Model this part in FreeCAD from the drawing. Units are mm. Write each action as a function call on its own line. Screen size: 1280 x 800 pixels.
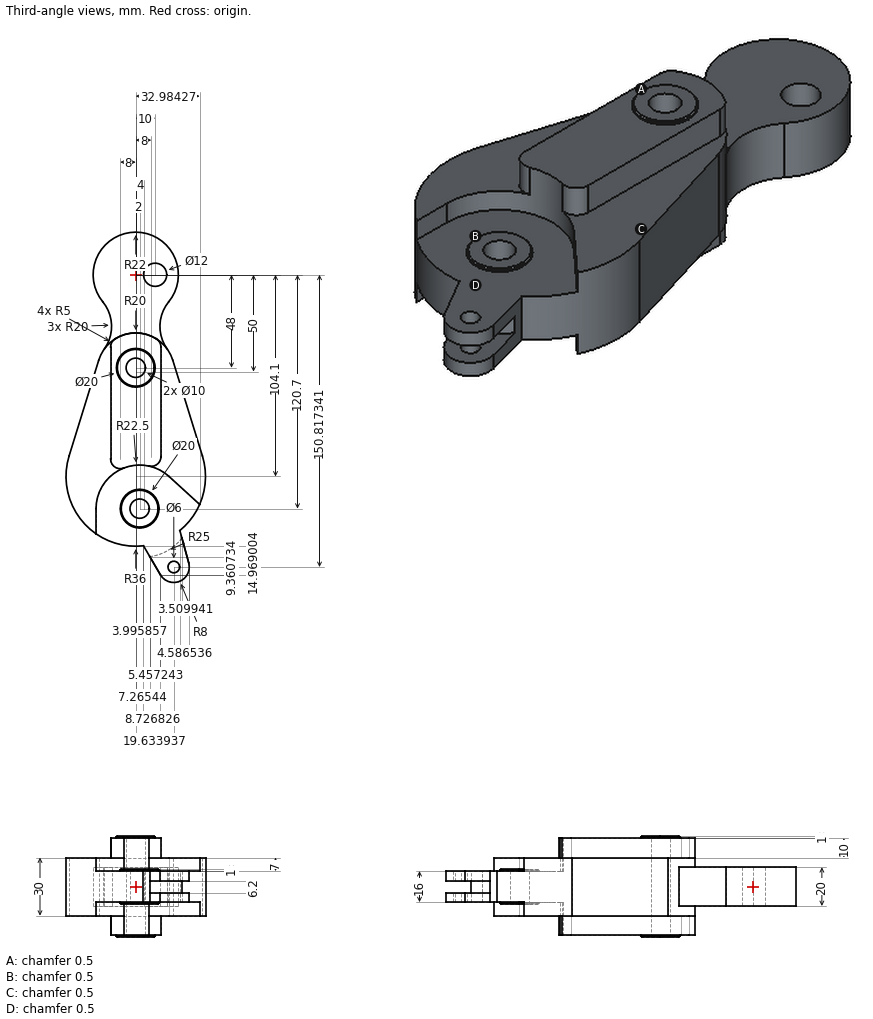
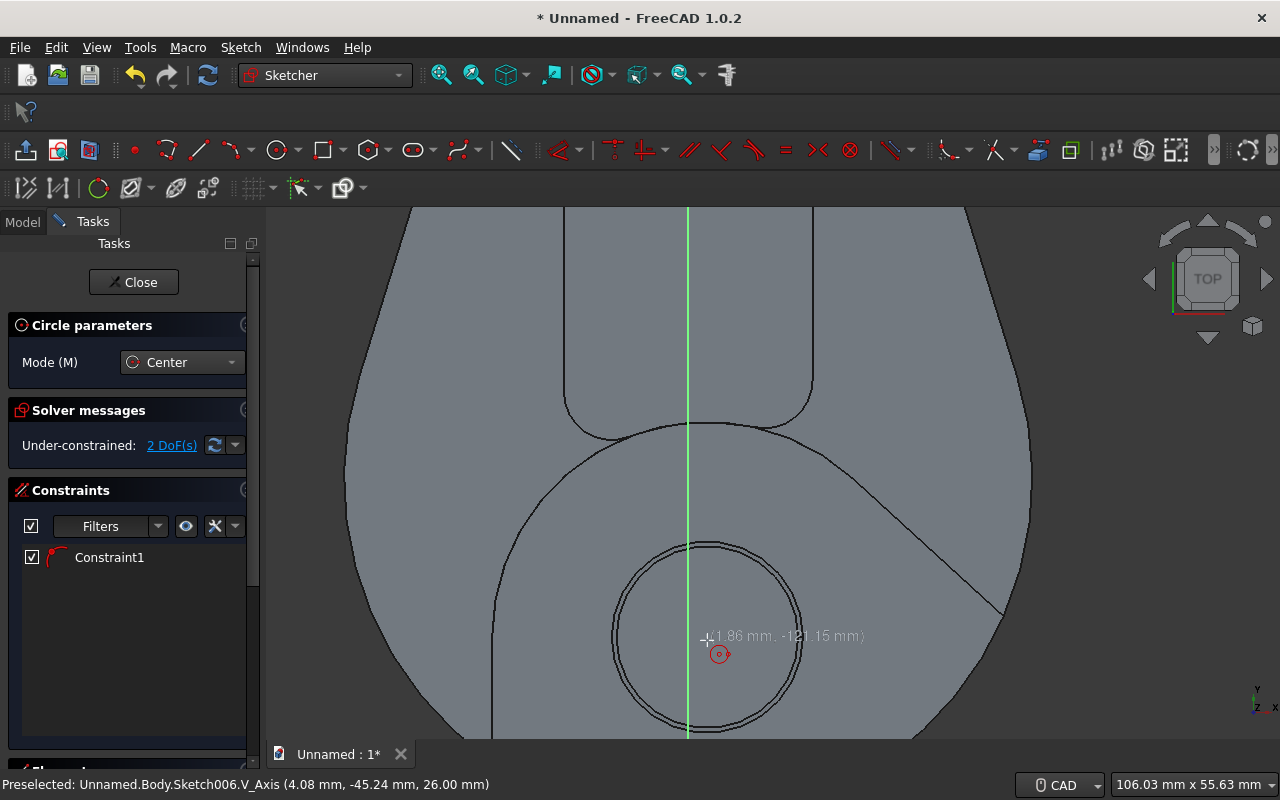
click(707, 637)
click(741, 603)
key(Escape)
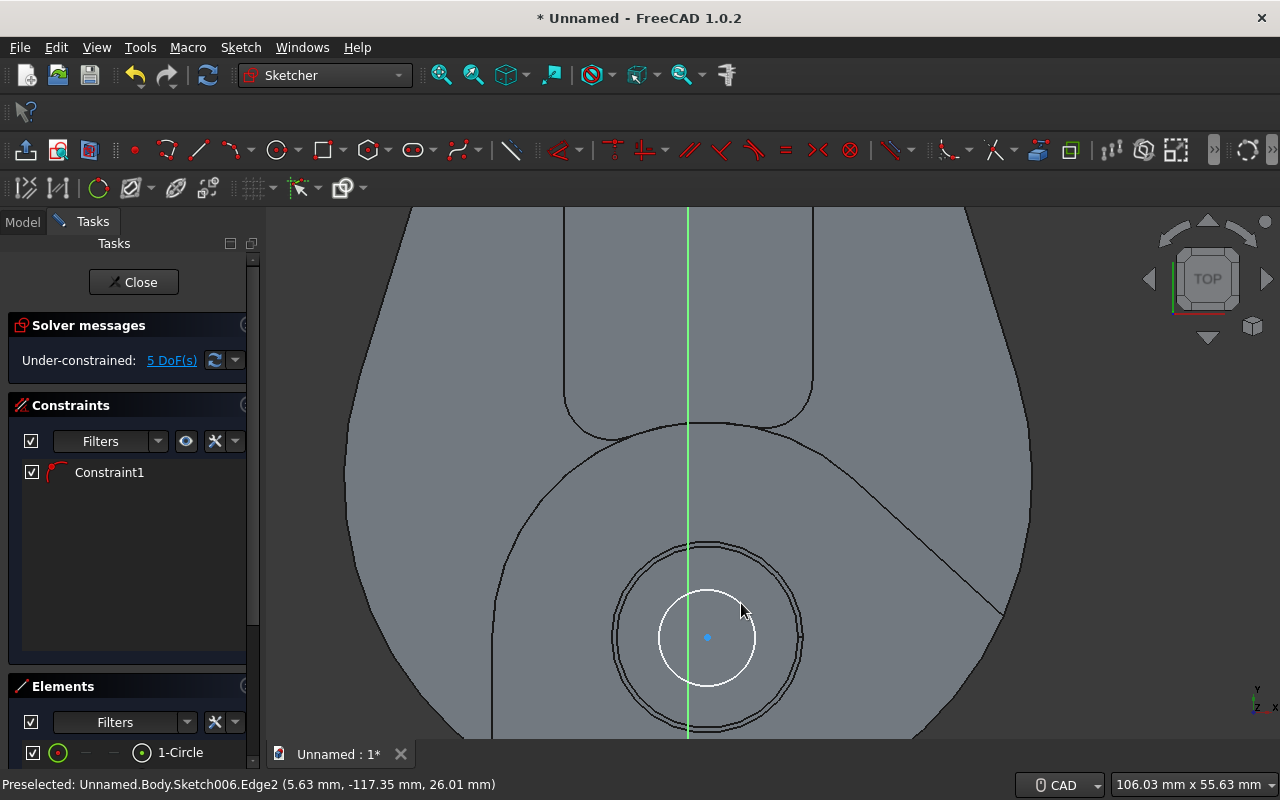
scroll(707, 641, down, 6)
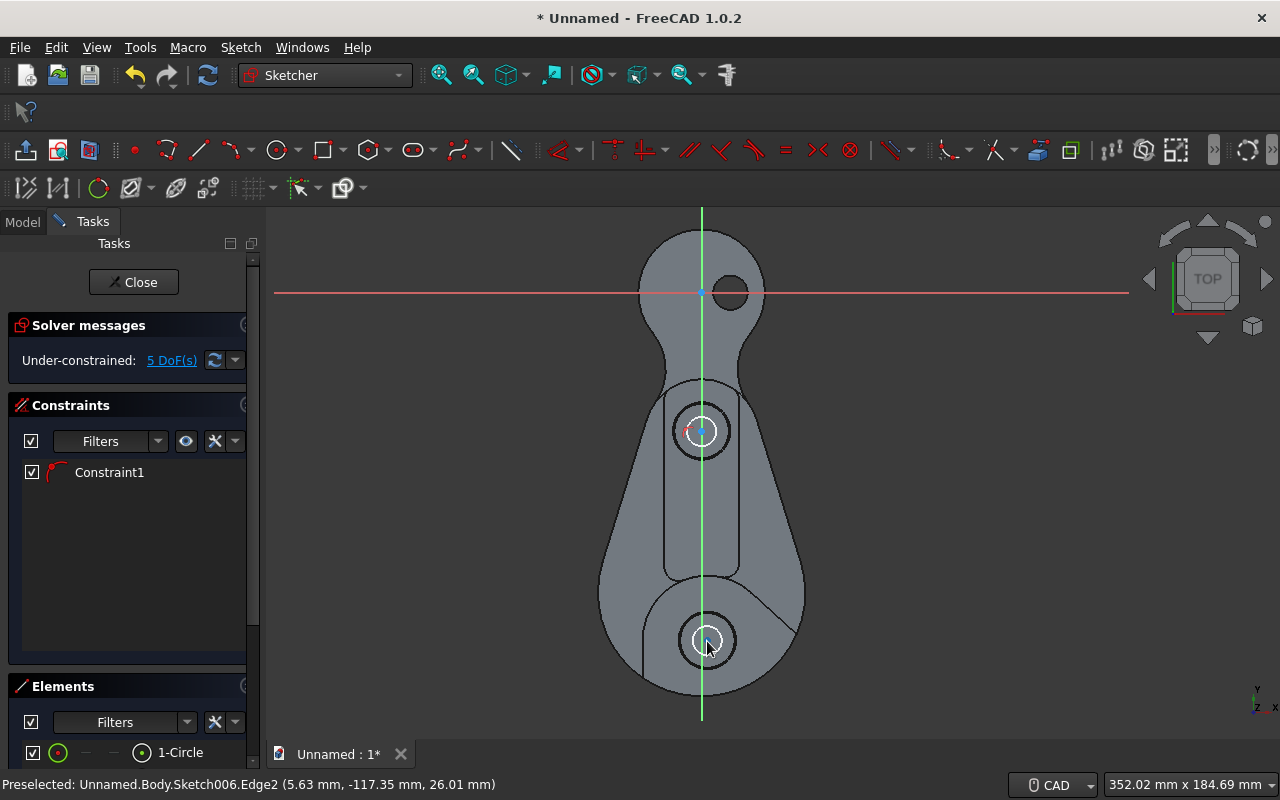
scroll(712, 421, up, 2)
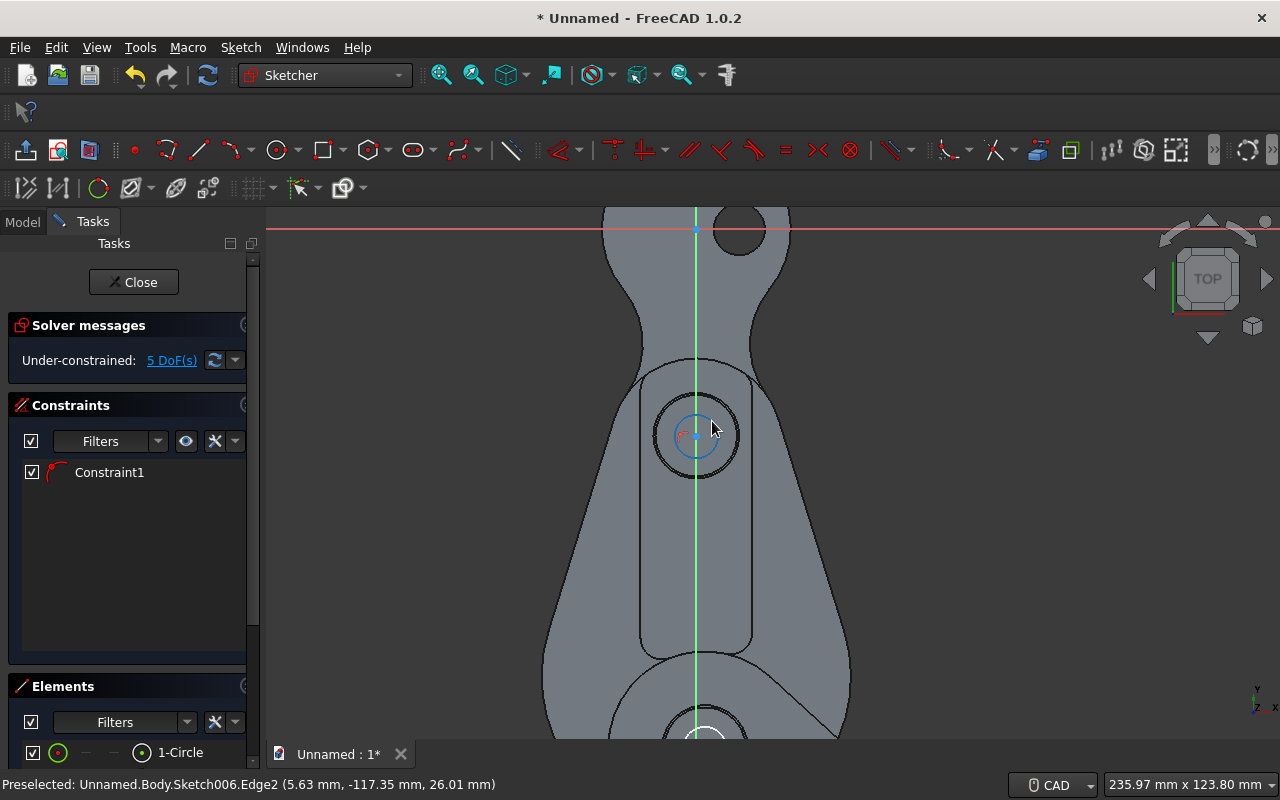
click(712, 421)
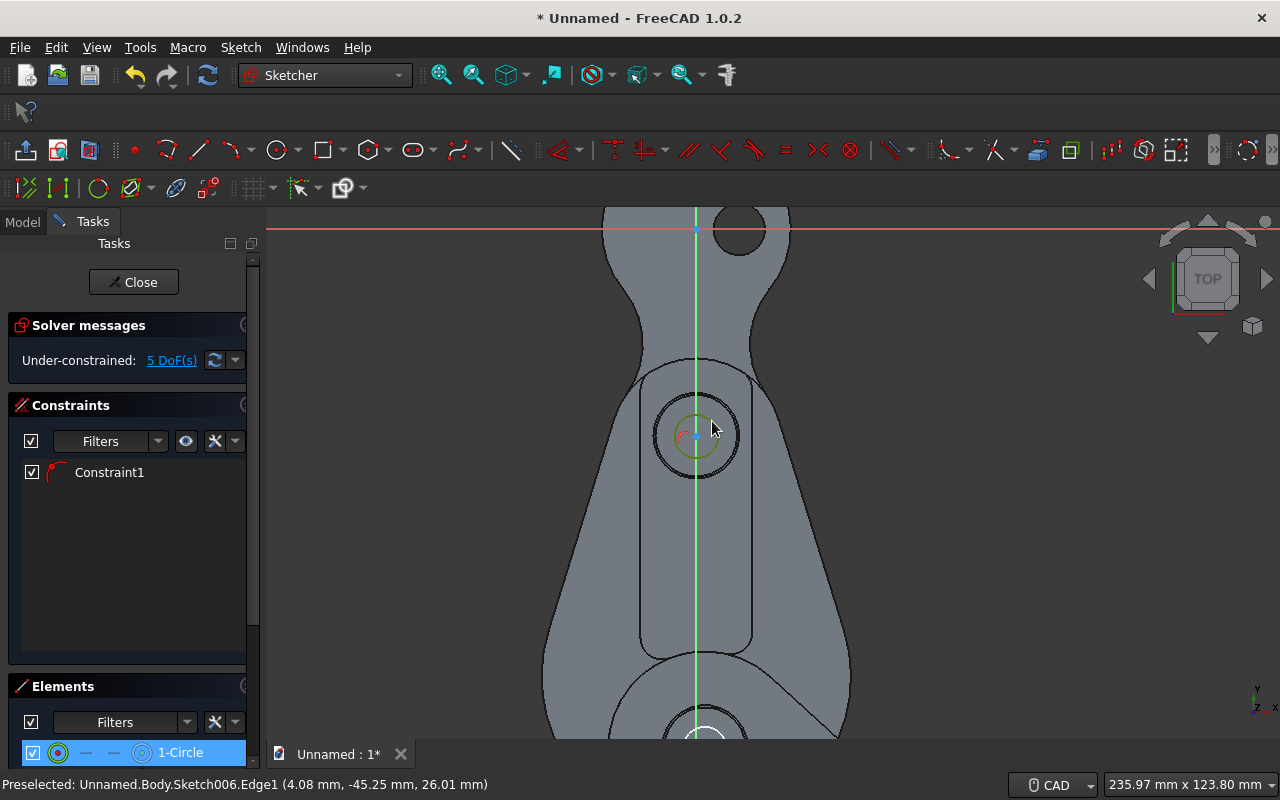
scroll(712, 419, down, 2)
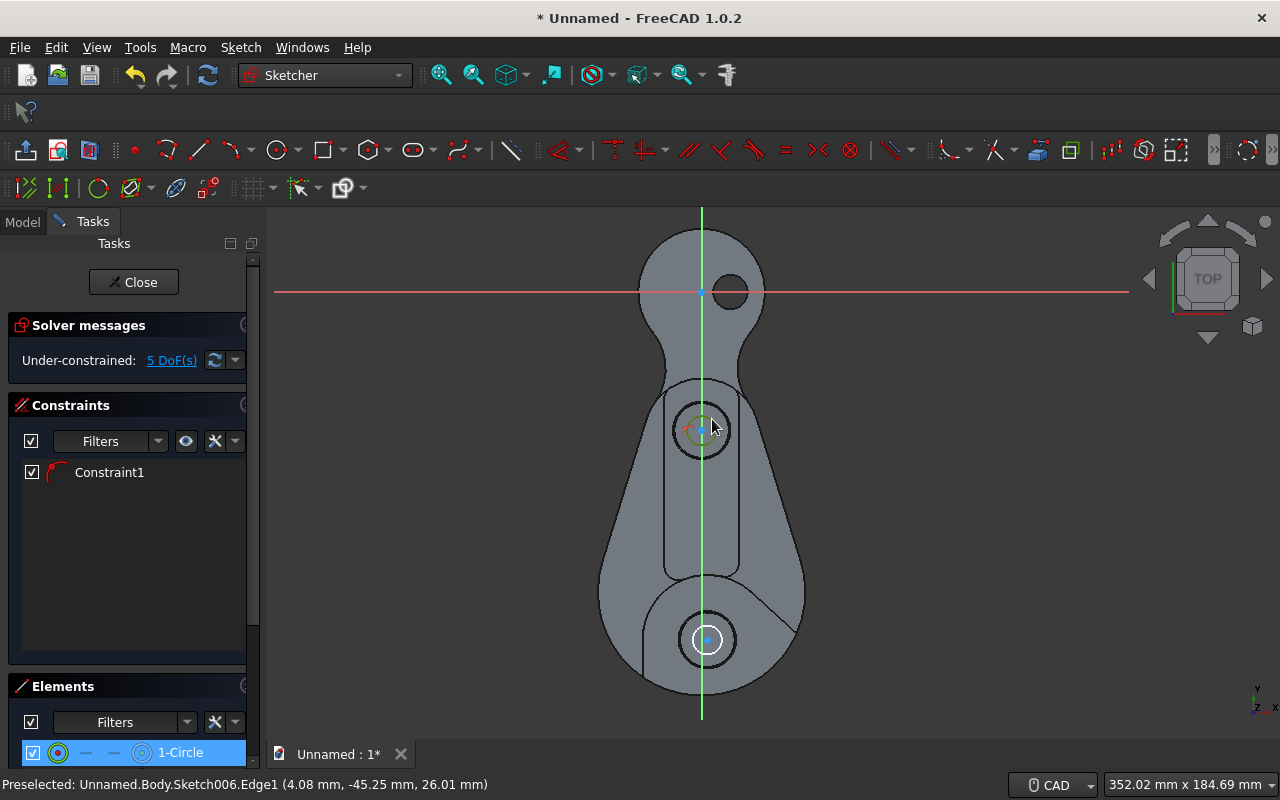
click(718, 630)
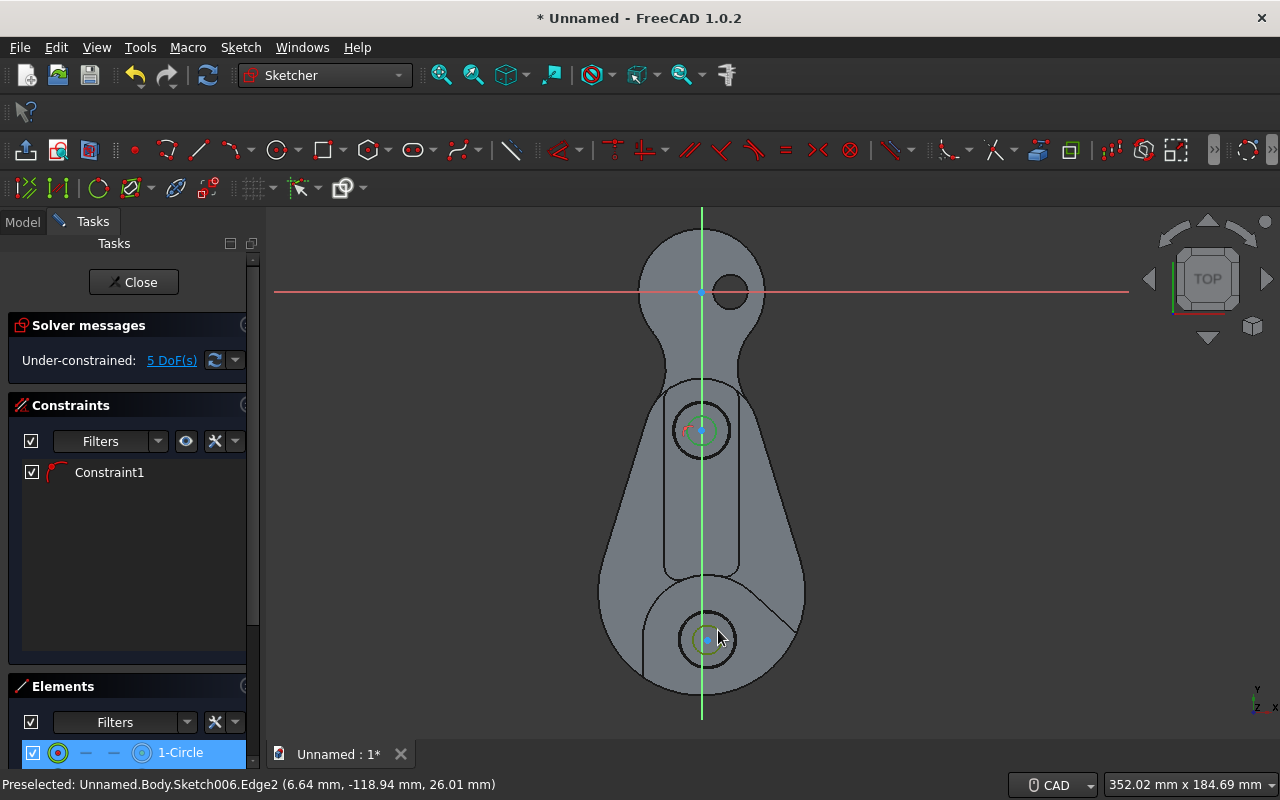
click(786, 150)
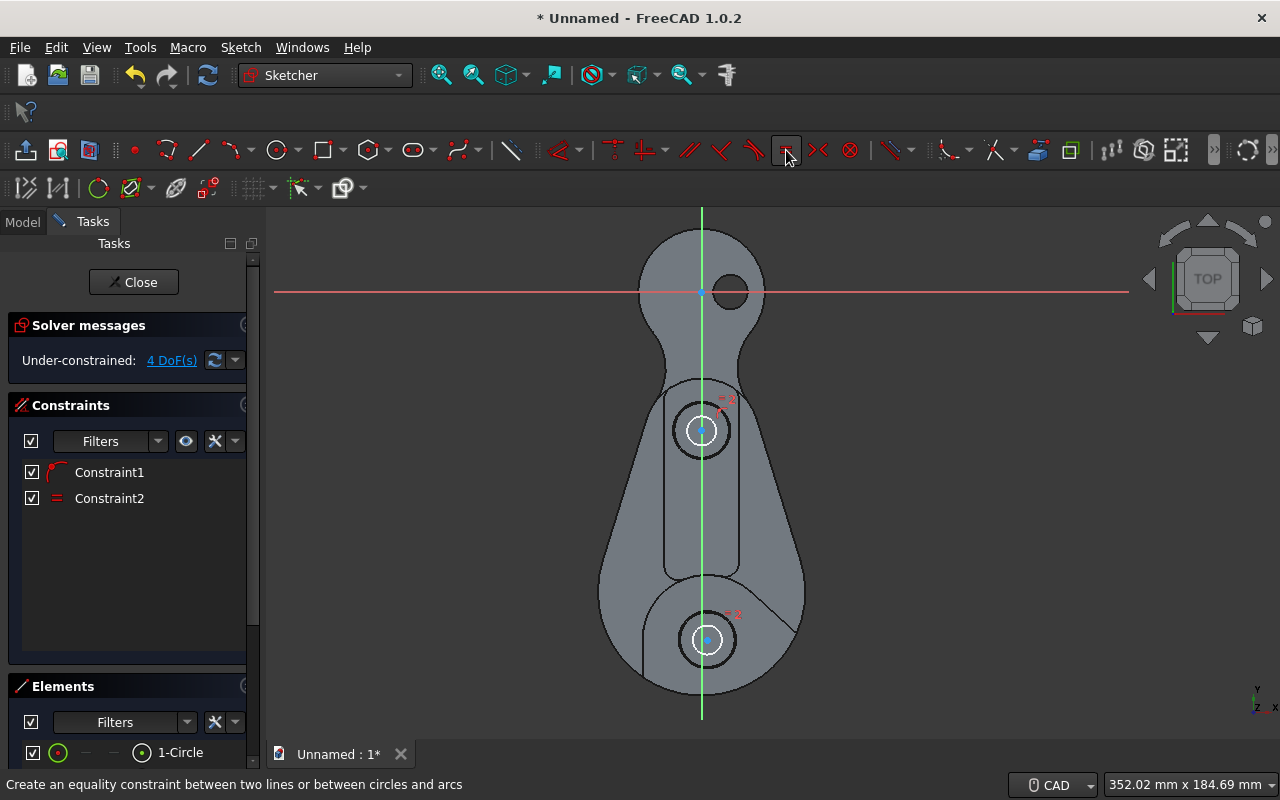
click(558, 150)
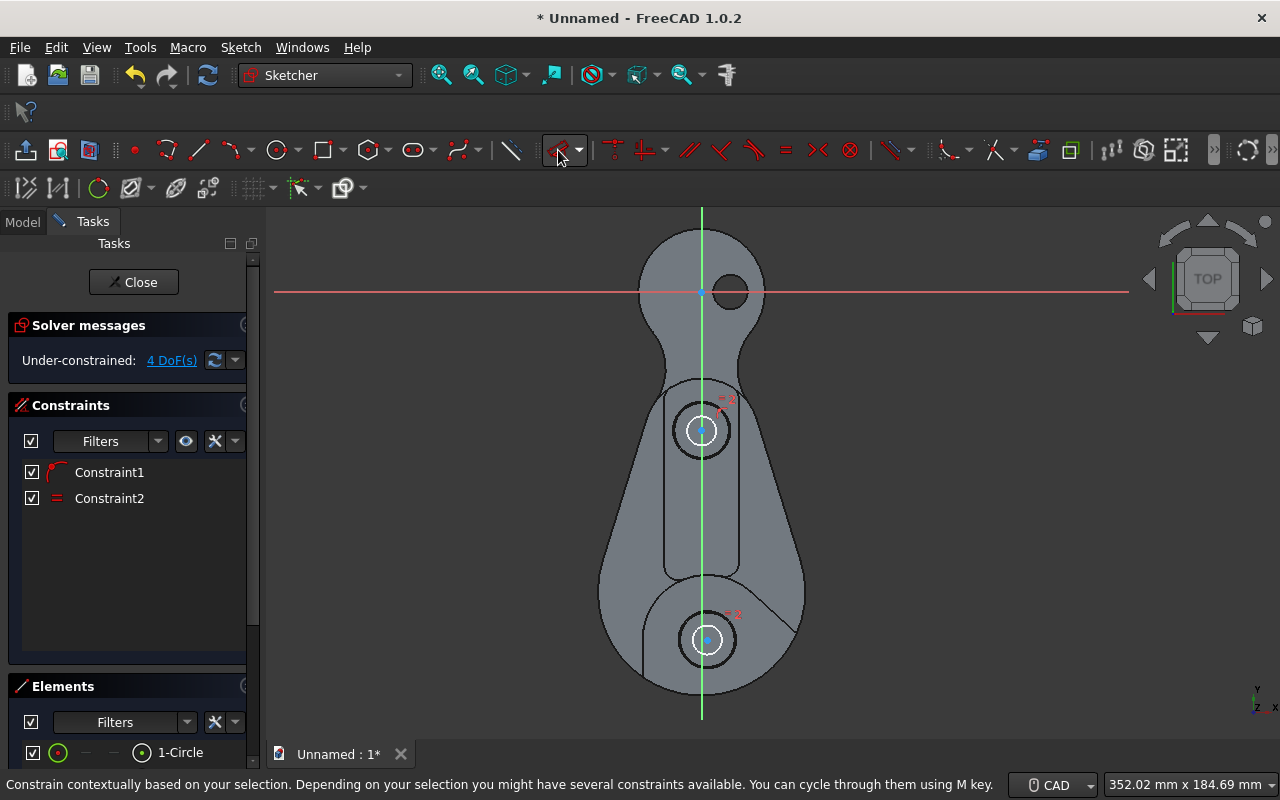
scroll(712, 421, up, 2)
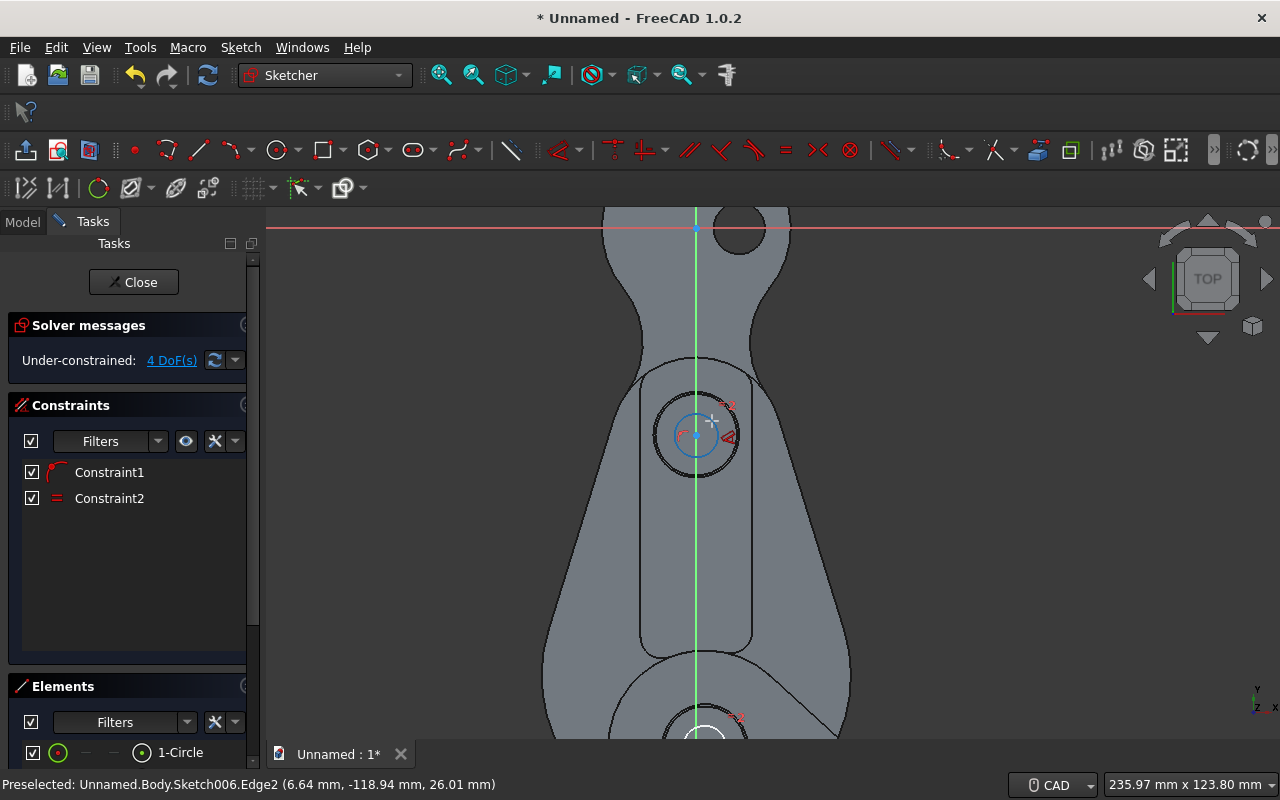
click(712, 420)
click(735, 397)